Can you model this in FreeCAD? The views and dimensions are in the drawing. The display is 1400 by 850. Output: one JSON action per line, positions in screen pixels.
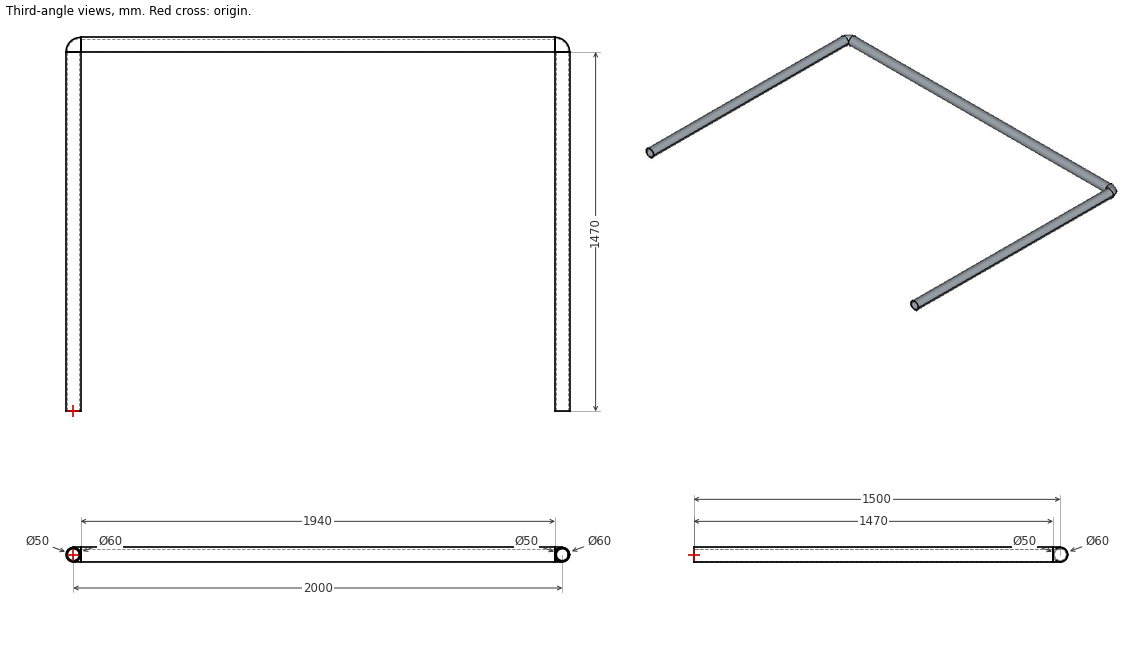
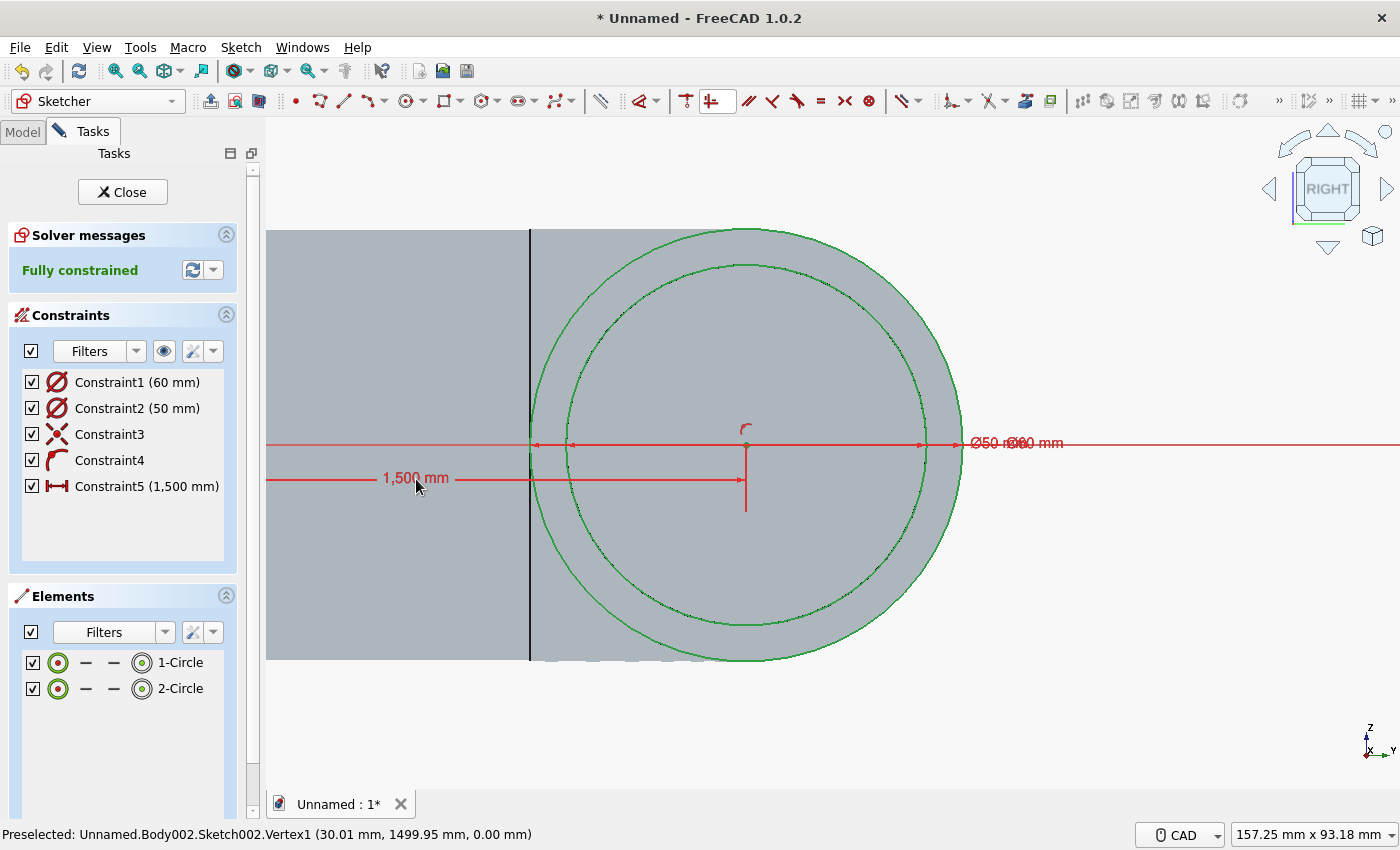
{"action": "left_click", "coordinate": [123, 192]}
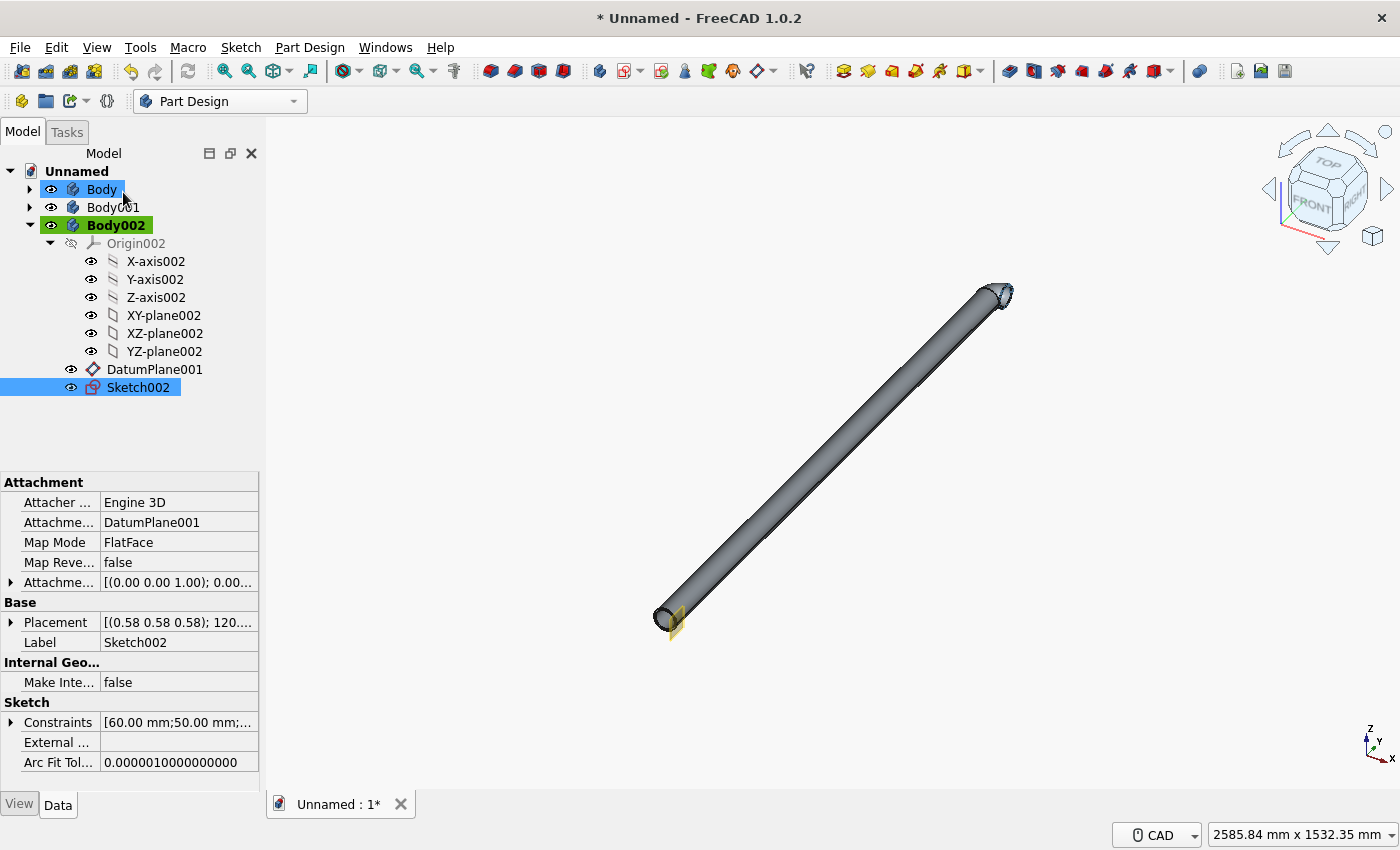
{"action": "left_click", "coordinate": [844, 72]}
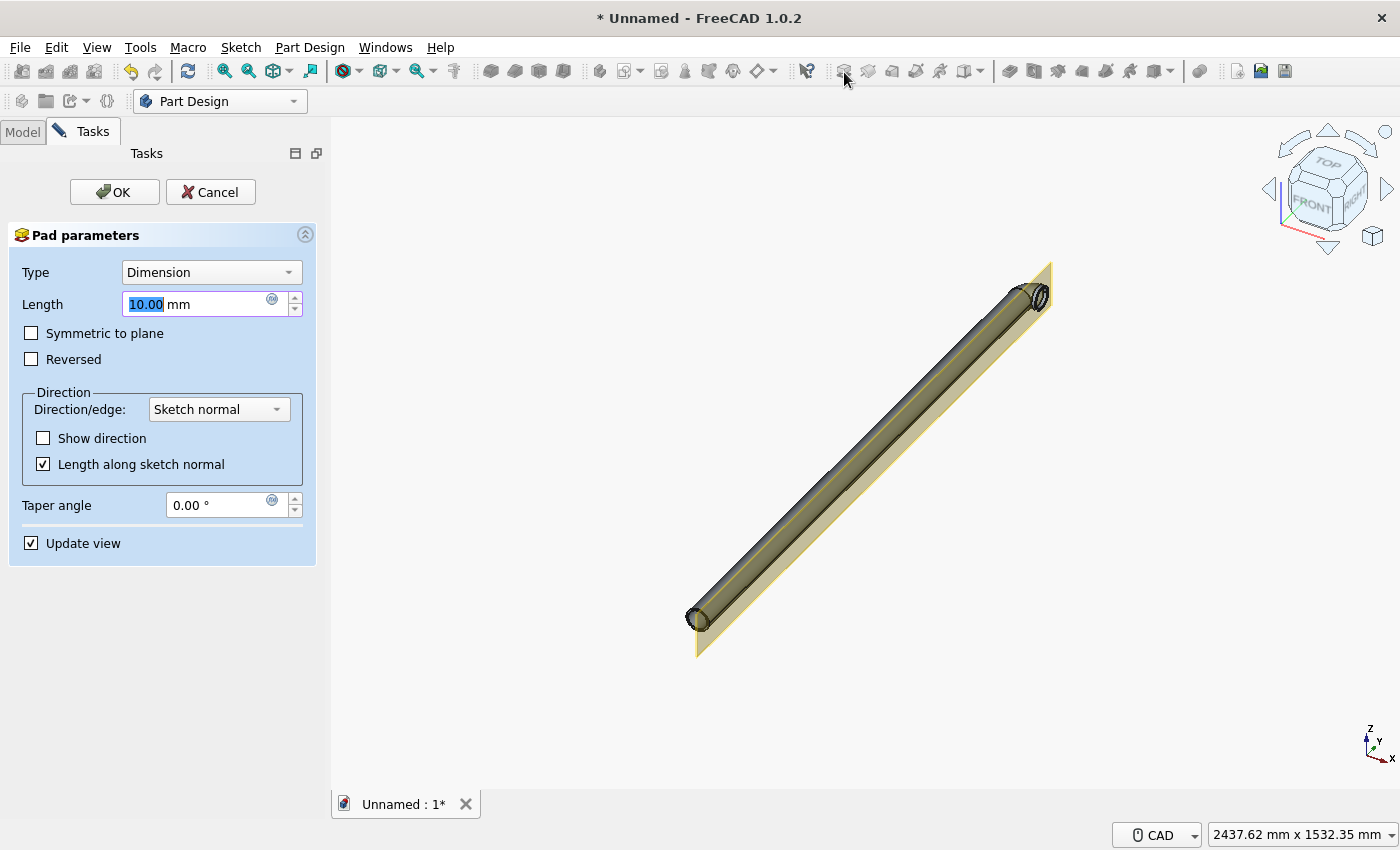
{"action": "type", "text": "1940"}
{"action": "key", "text": "Tab"}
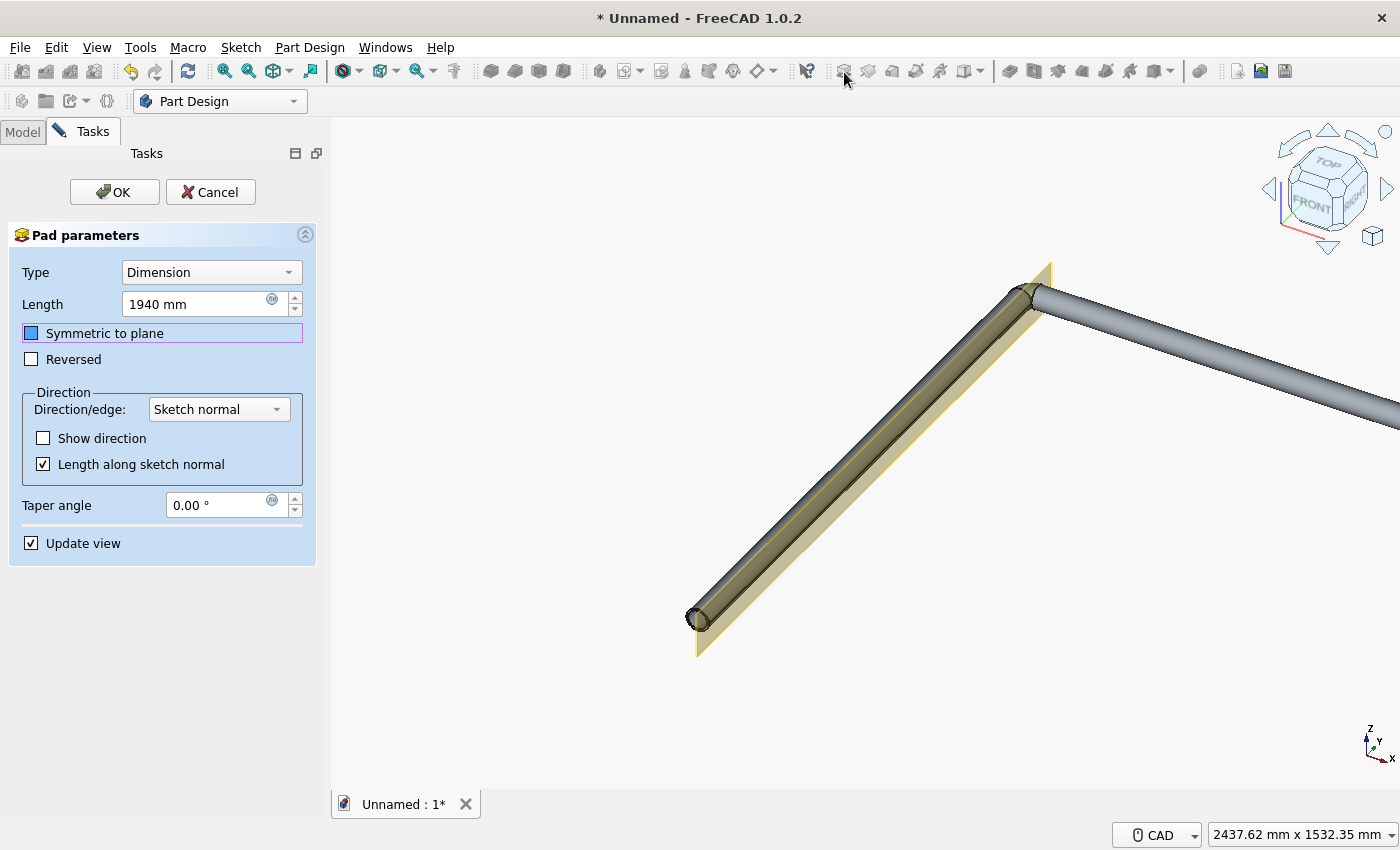
{"action": "left_click", "coordinate": [115, 192]}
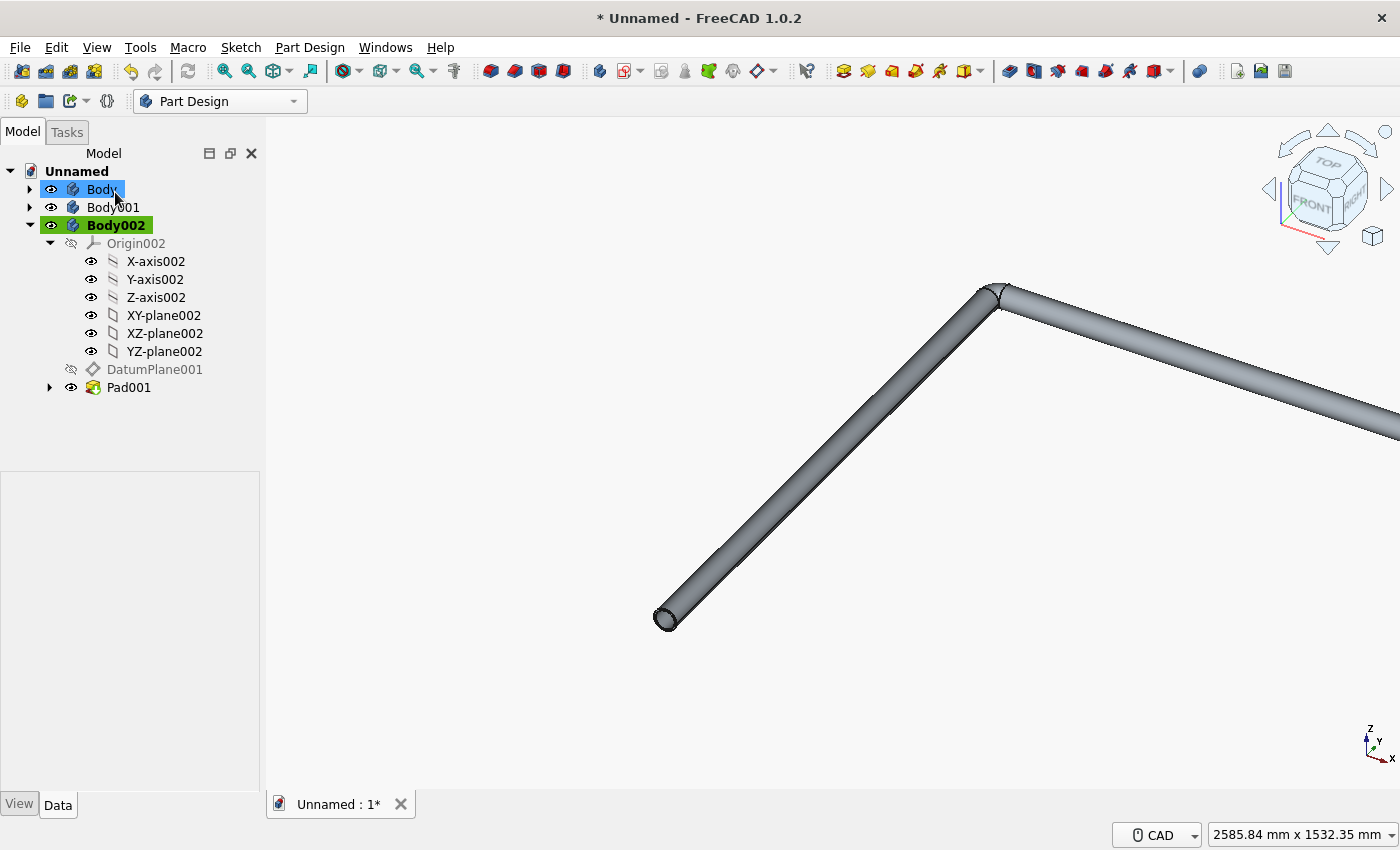
{"action": "left_click", "coordinate": [226, 72]}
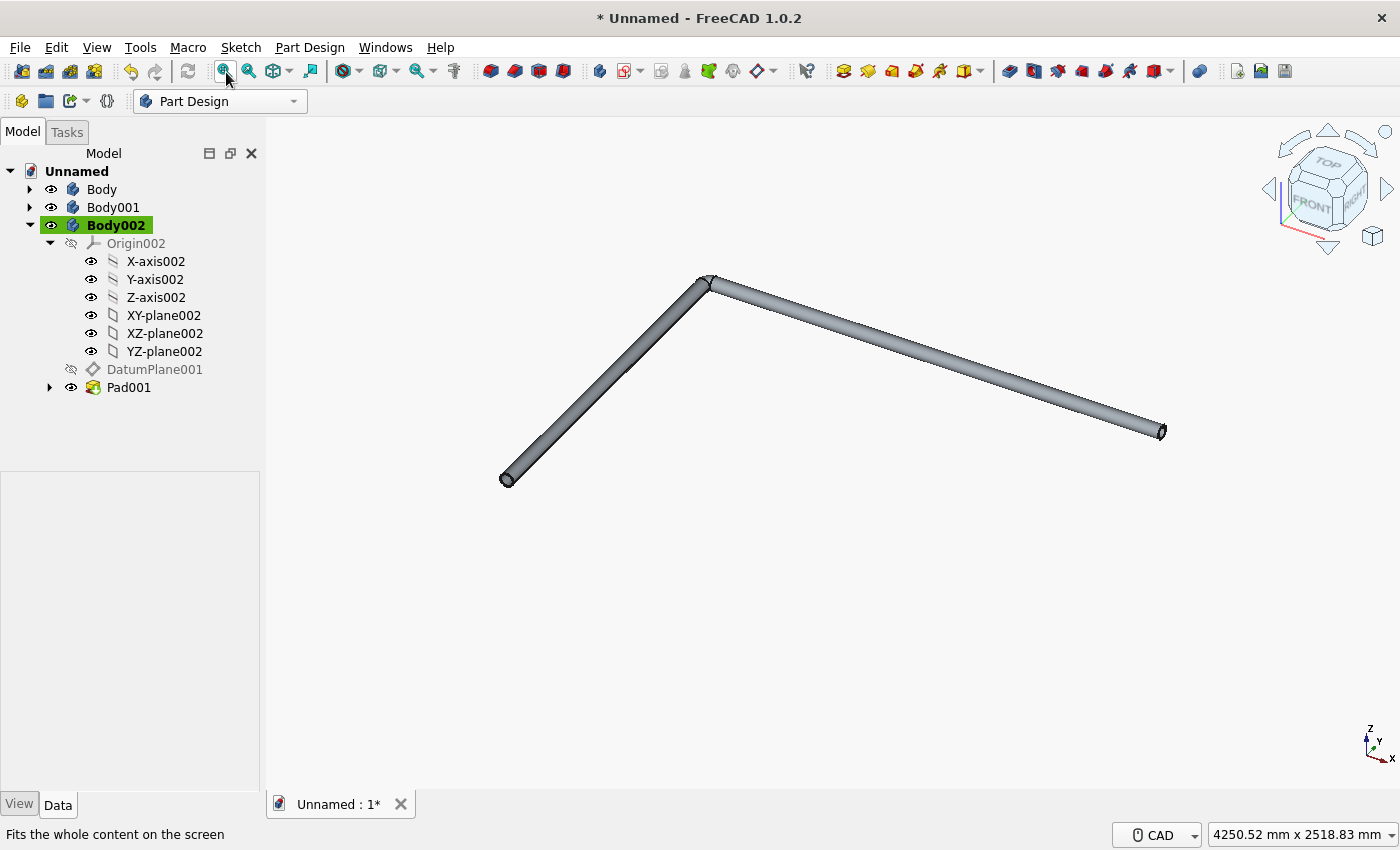
{"action": "left_click", "coordinate": [600, 72]}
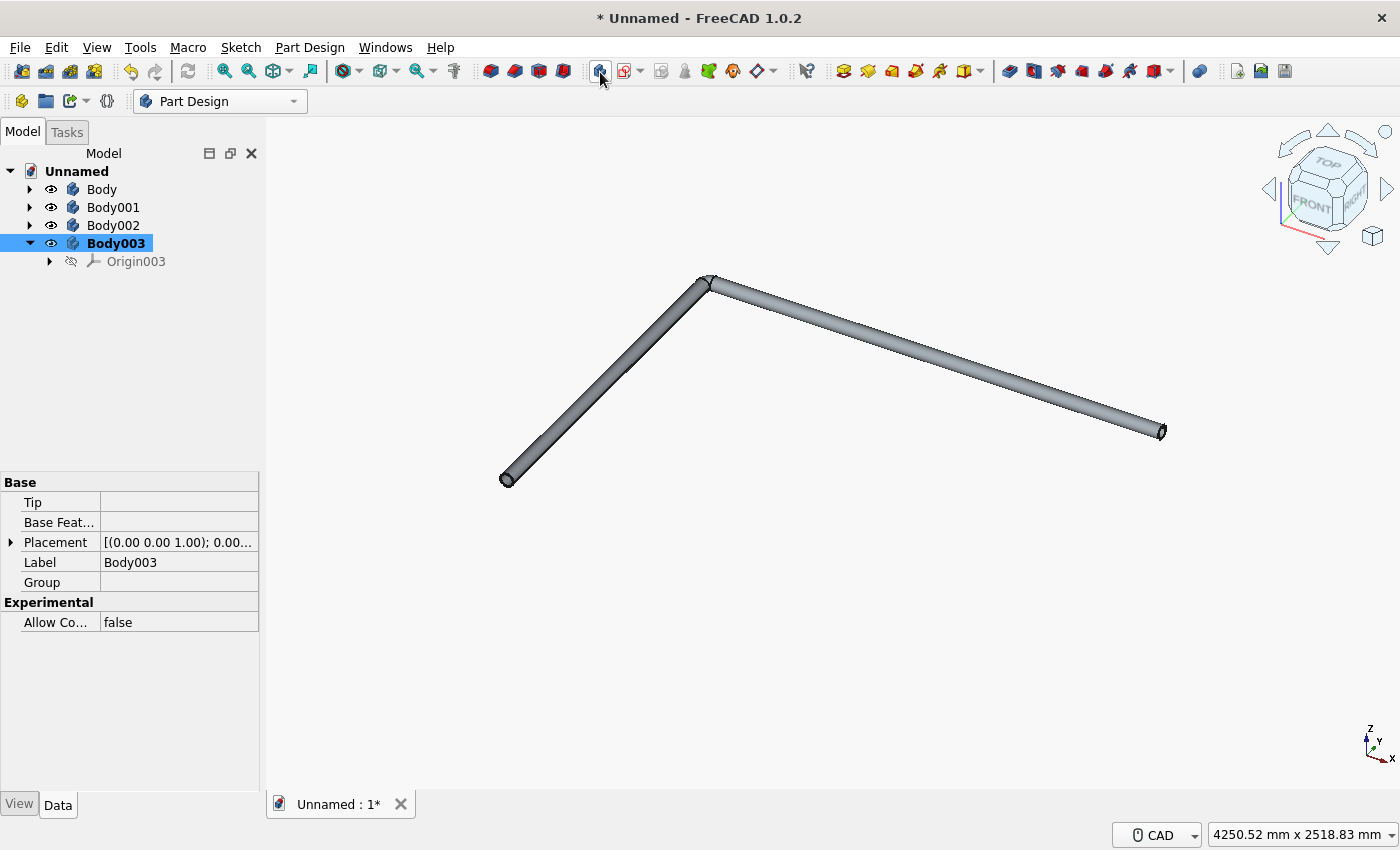
{"action": "left_click", "coordinate": [50, 261]}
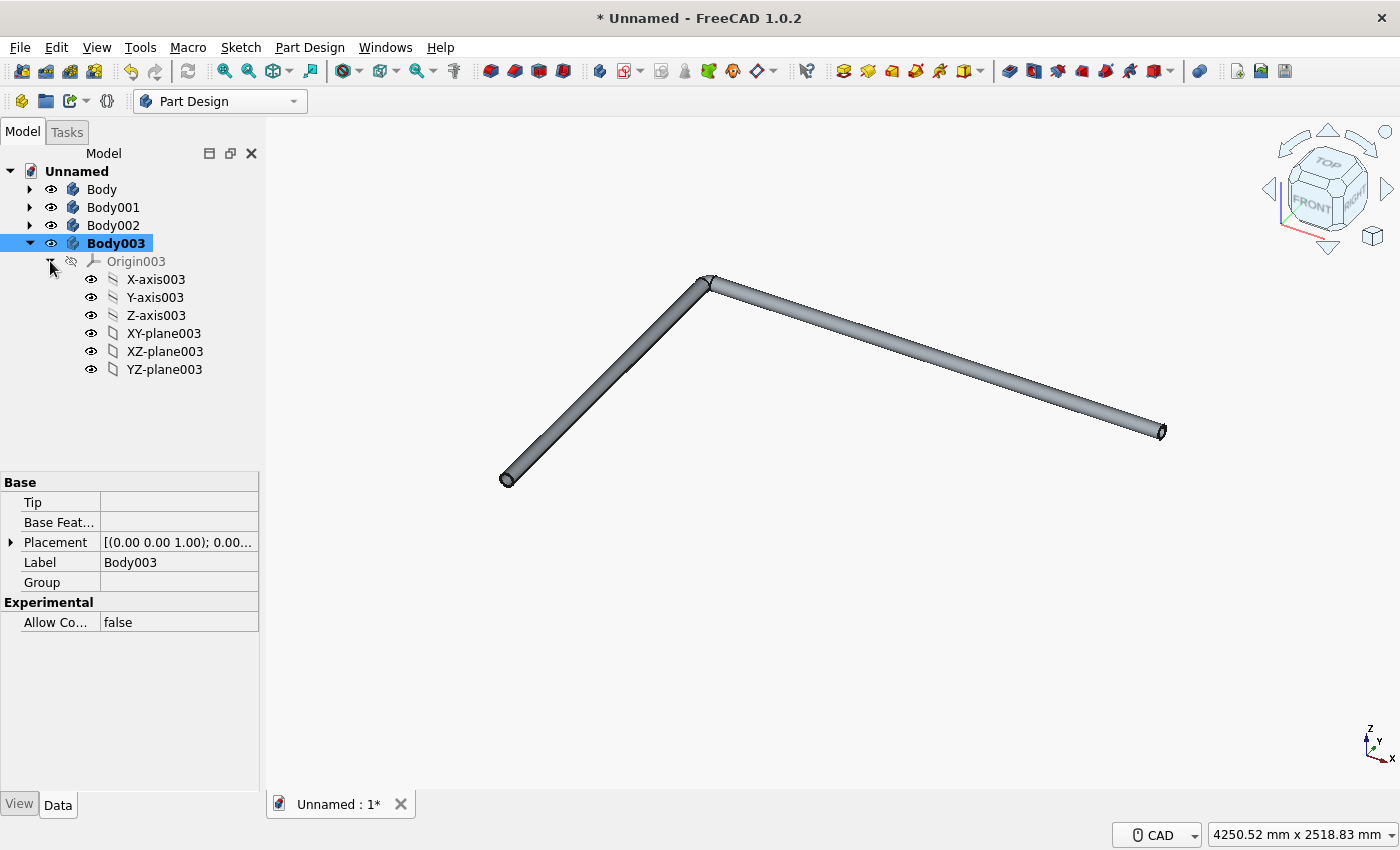
{"action": "left_click", "coordinate": [136, 351]}